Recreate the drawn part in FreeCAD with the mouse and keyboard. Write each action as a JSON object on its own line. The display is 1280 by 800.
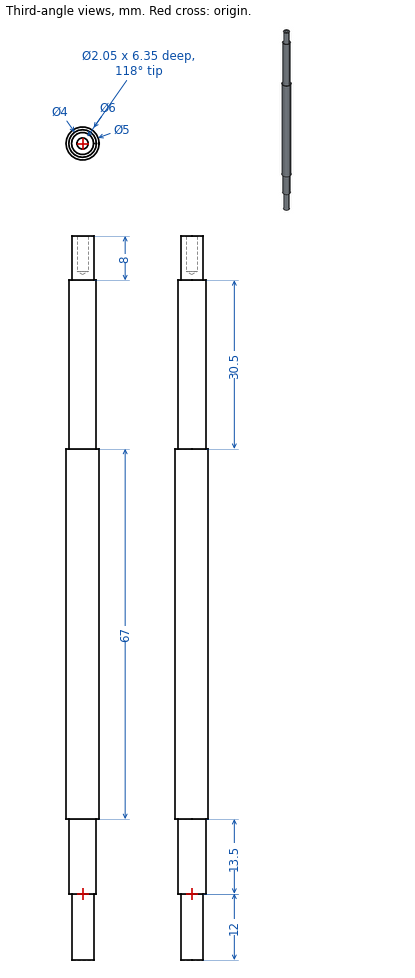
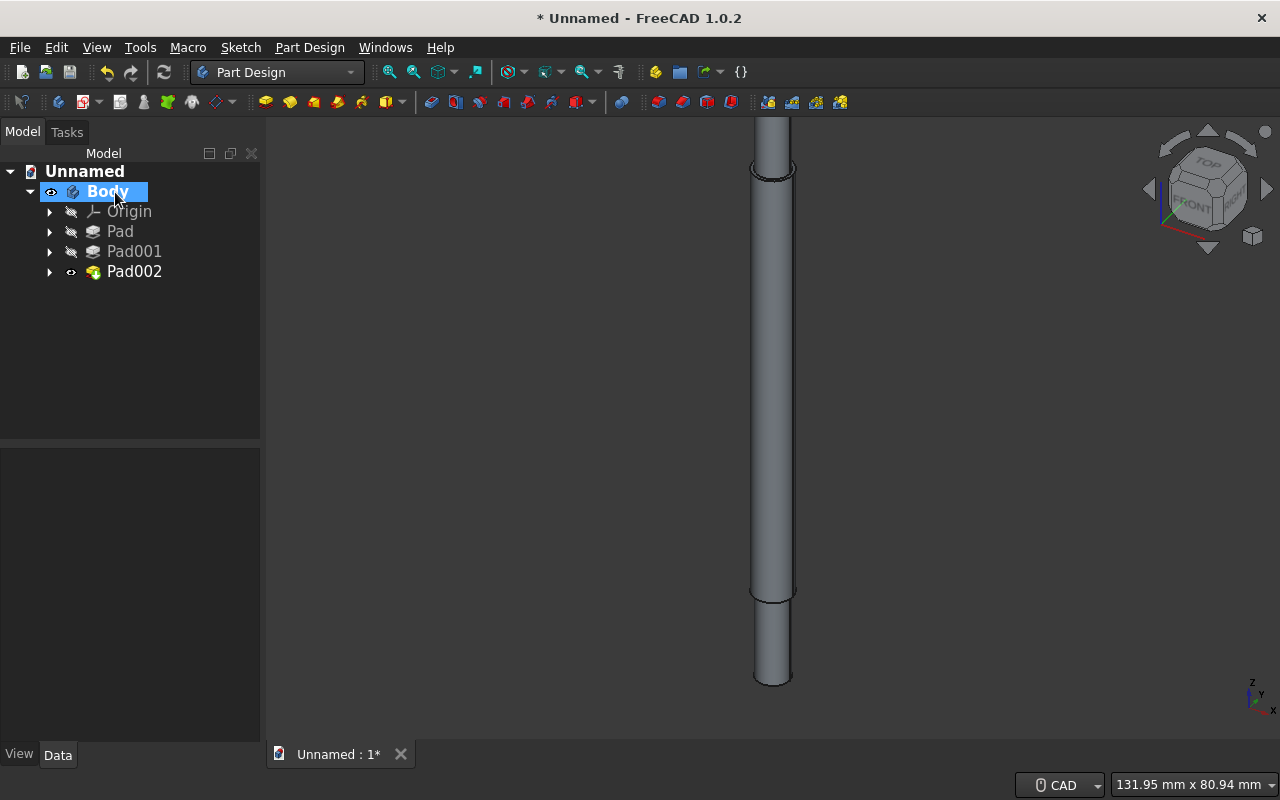
{"action": "left_click", "coordinate": [390, 72]}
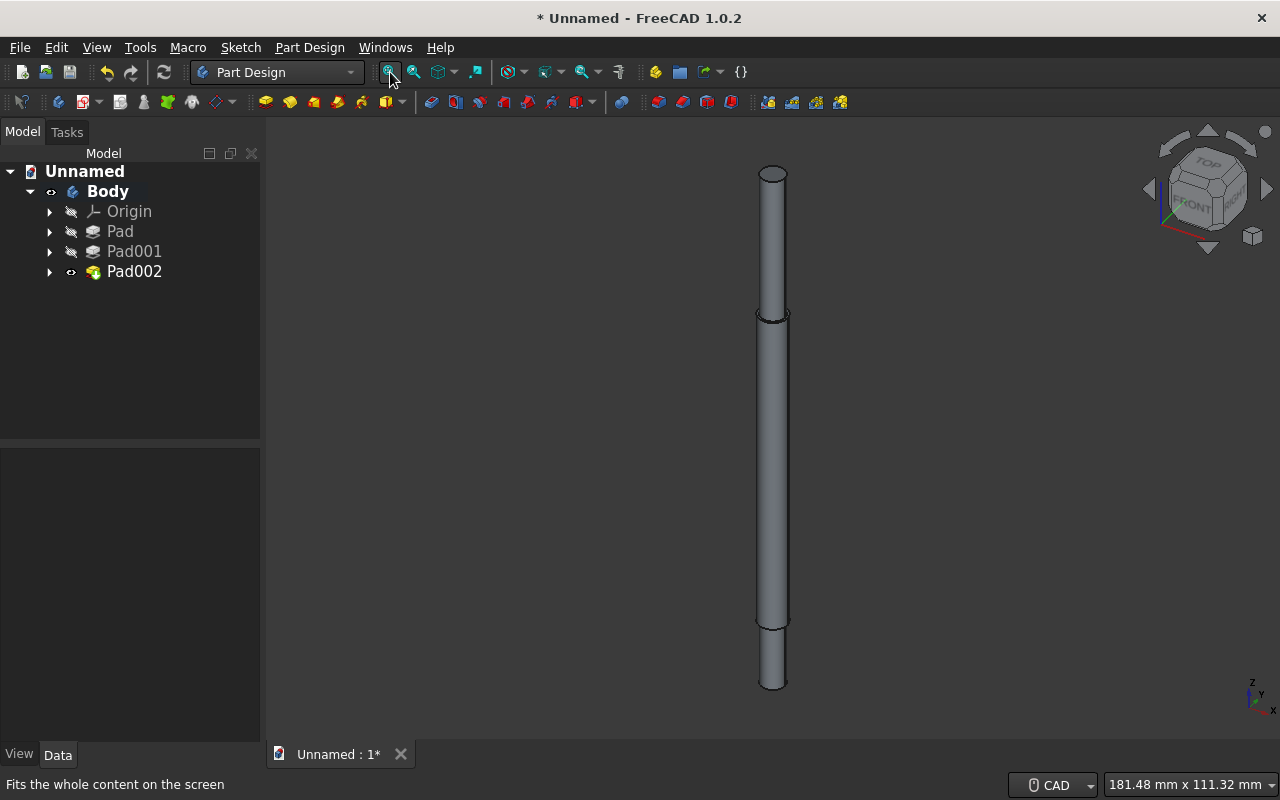
{"action": "left_click", "coordinate": [775, 171]}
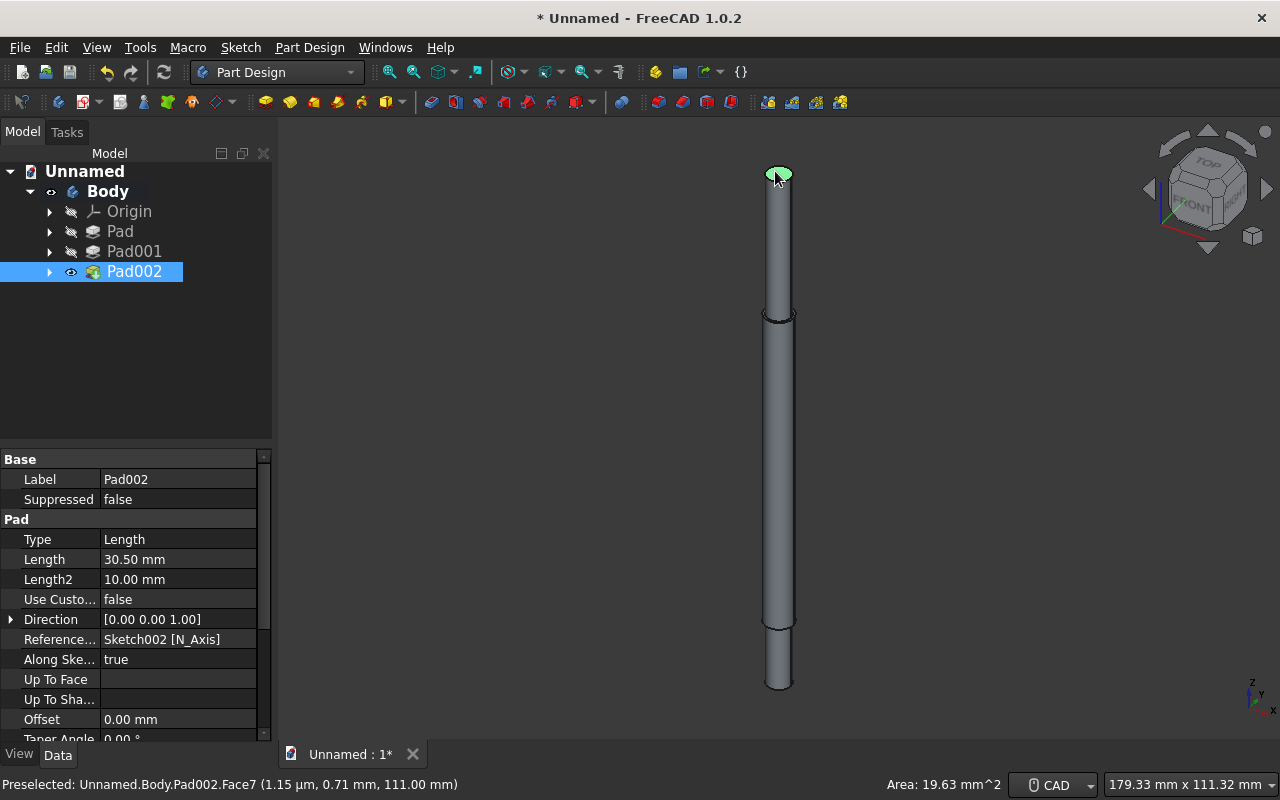
{"action": "left_click", "coordinate": [84, 102]}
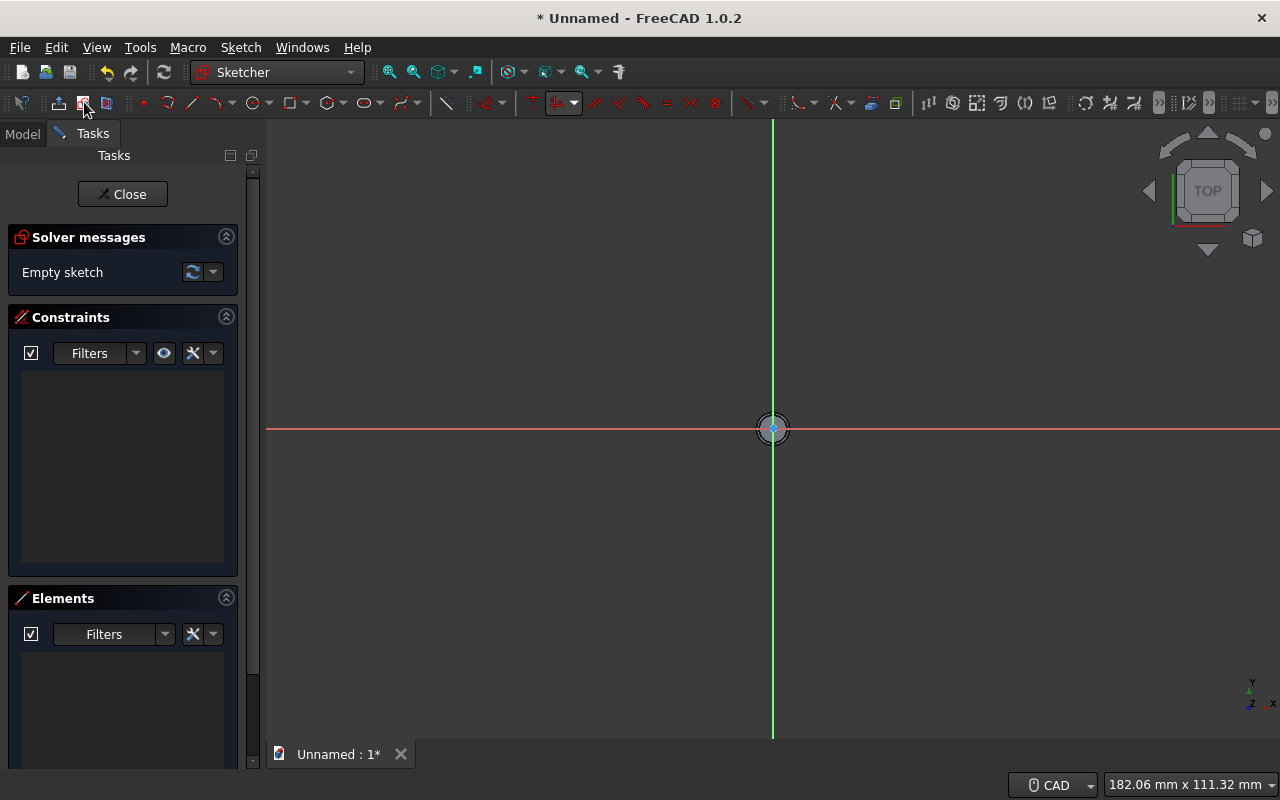
{"action": "scroll", "coordinate": [777, 429], "scroll_direction": "up", "scroll_amount": 14}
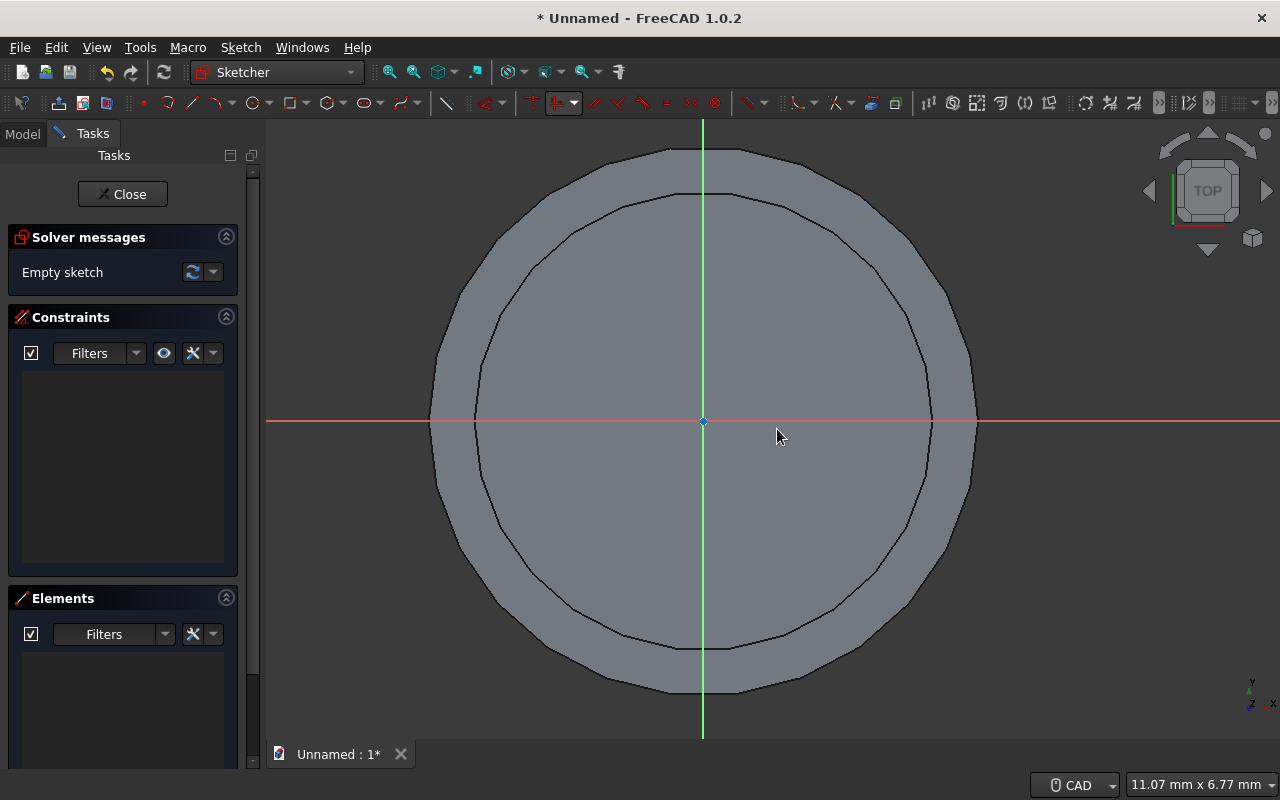
{"action": "key", "text": "g c"}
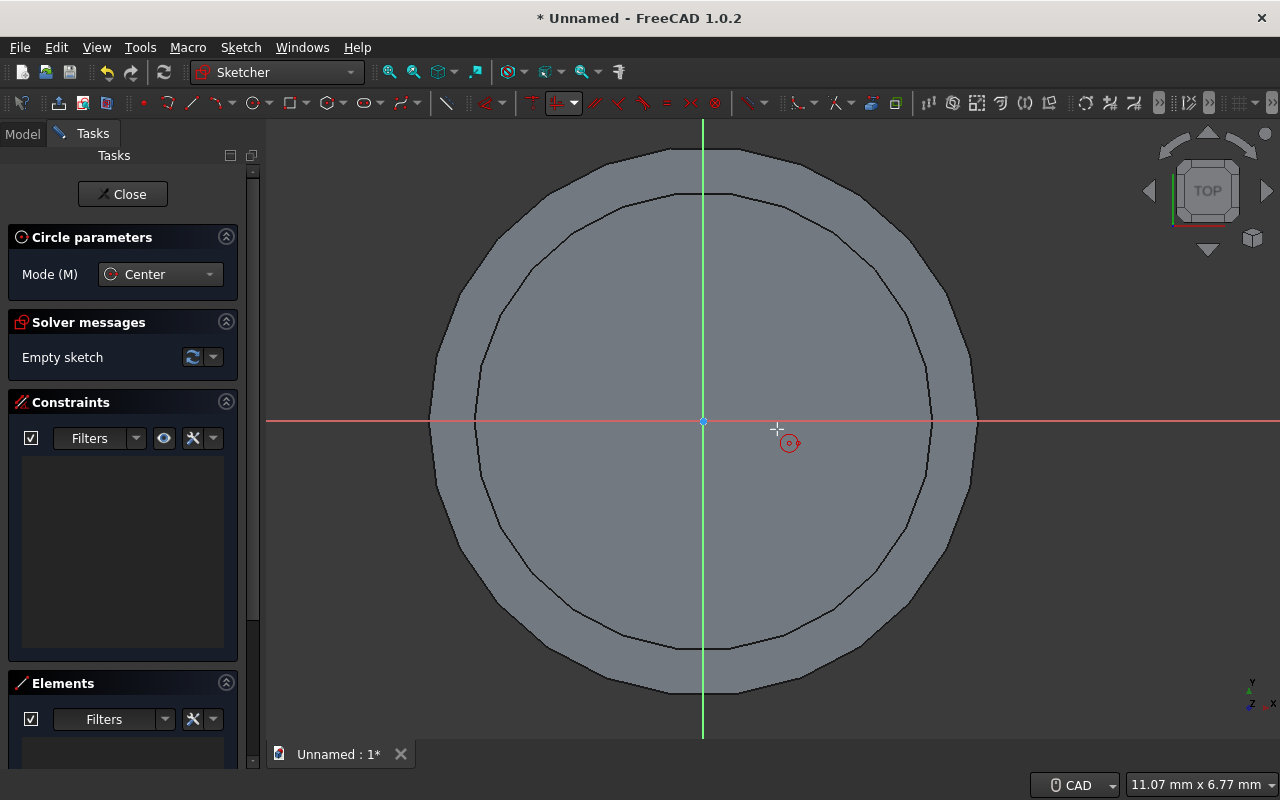
{"action": "left_click", "coordinate": [703, 421]}
{"action": "left_click", "coordinate": [833, 292]}
{"action": "key", "text": "Escape"}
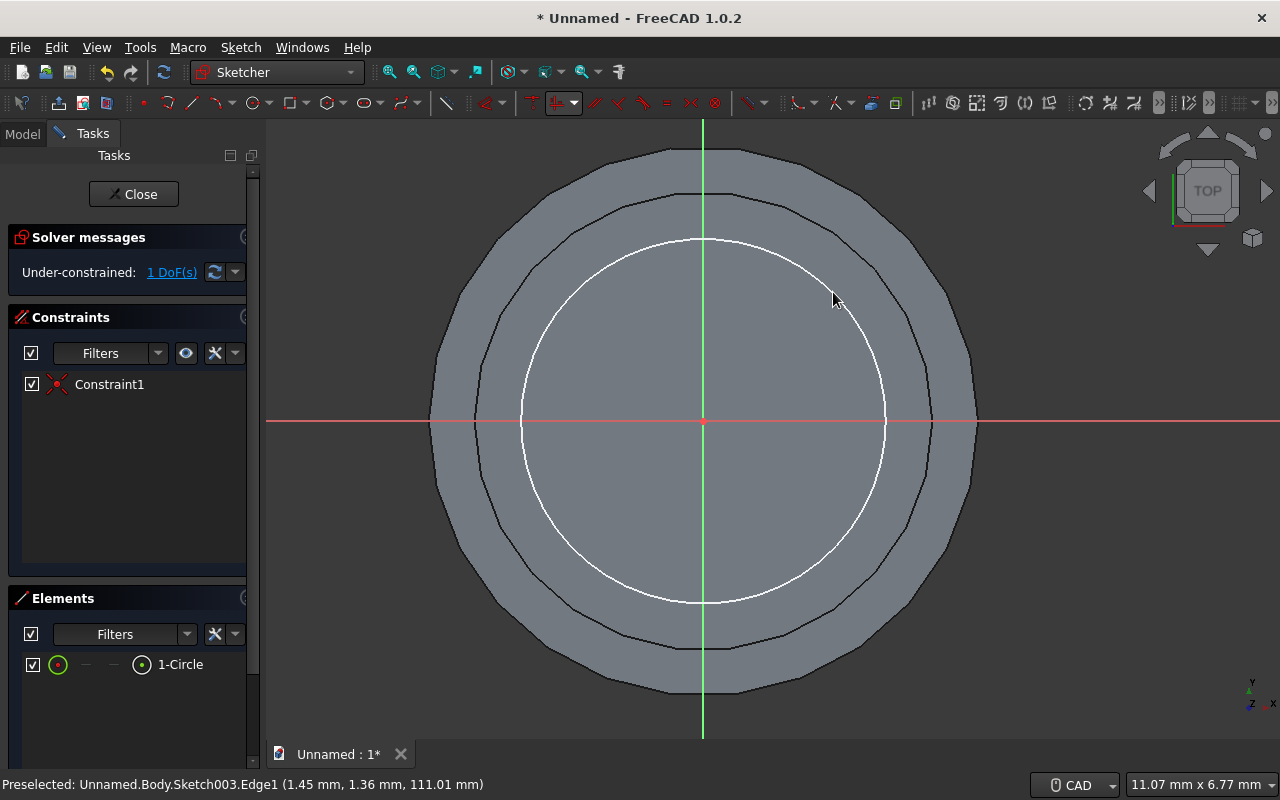
{"action": "left_click", "coordinate": [486, 104]}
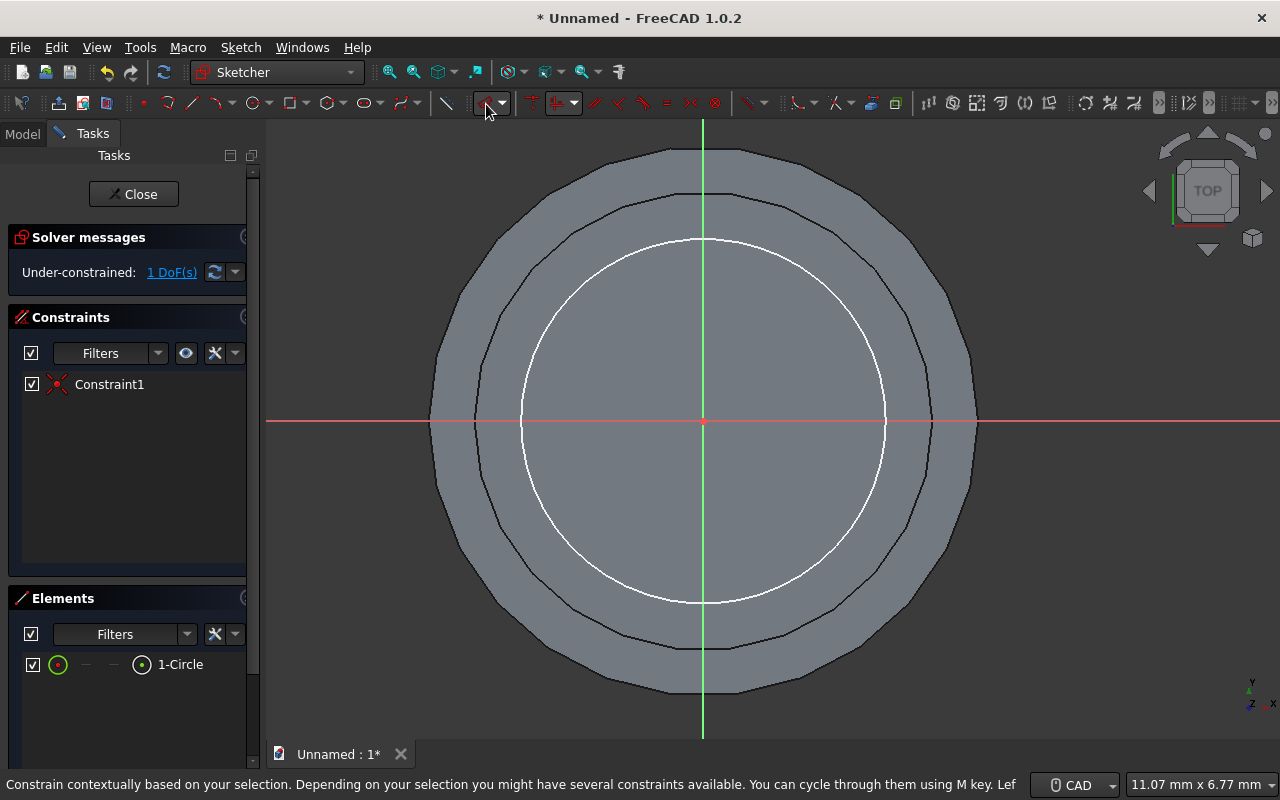
{"action": "left_click", "coordinate": [832, 292]}
{"action": "left_click", "coordinate": [855, 269]}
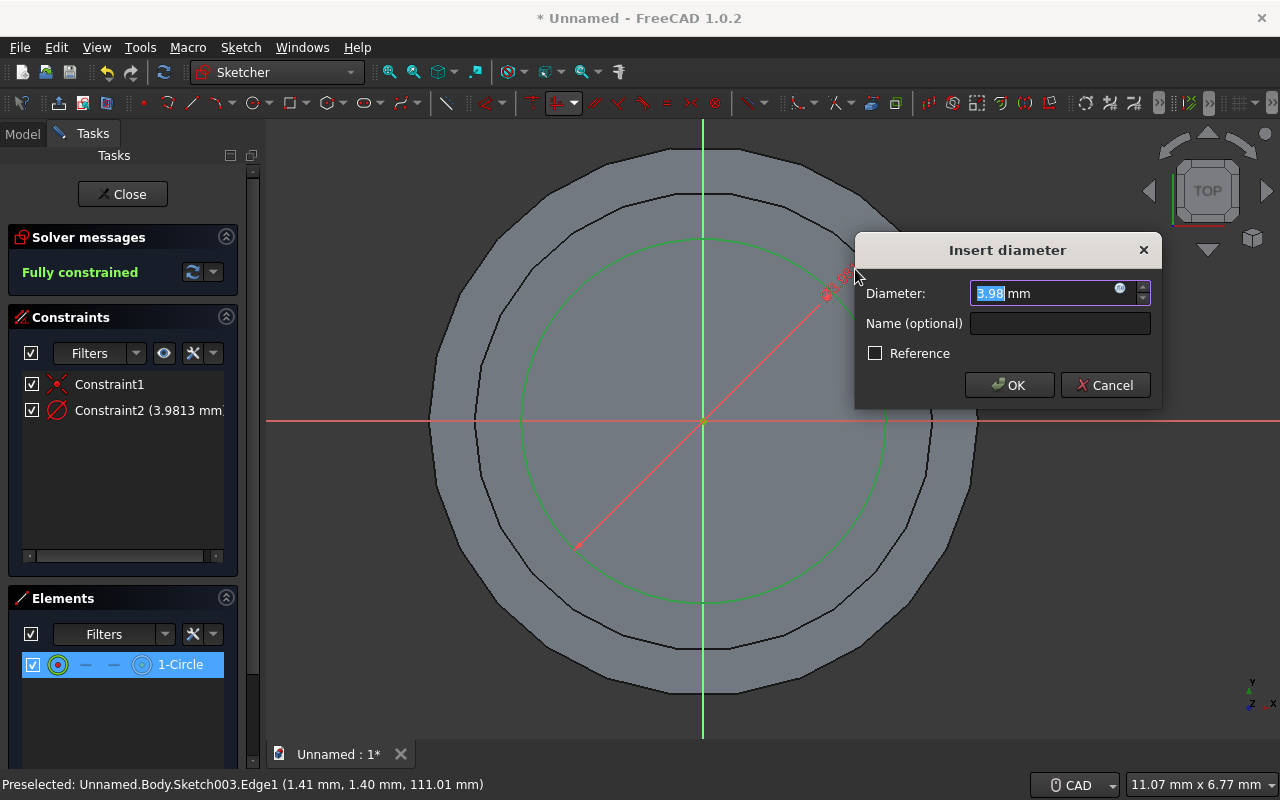
{"action": "type", "text": "4"}
{"action": "key", "text": "Return"}
{"action": "key", "text": "Escape"}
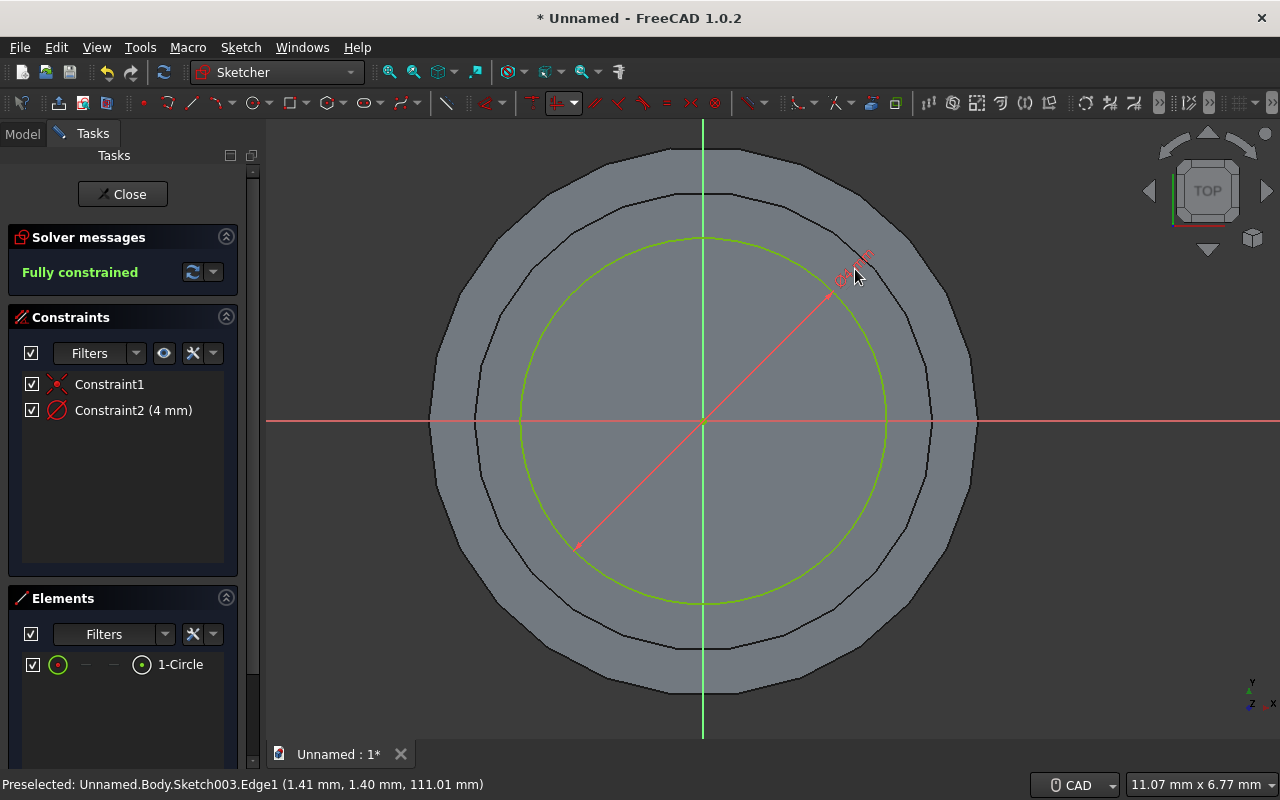
{"action": "left_click", "coordinate": [123, 194]}